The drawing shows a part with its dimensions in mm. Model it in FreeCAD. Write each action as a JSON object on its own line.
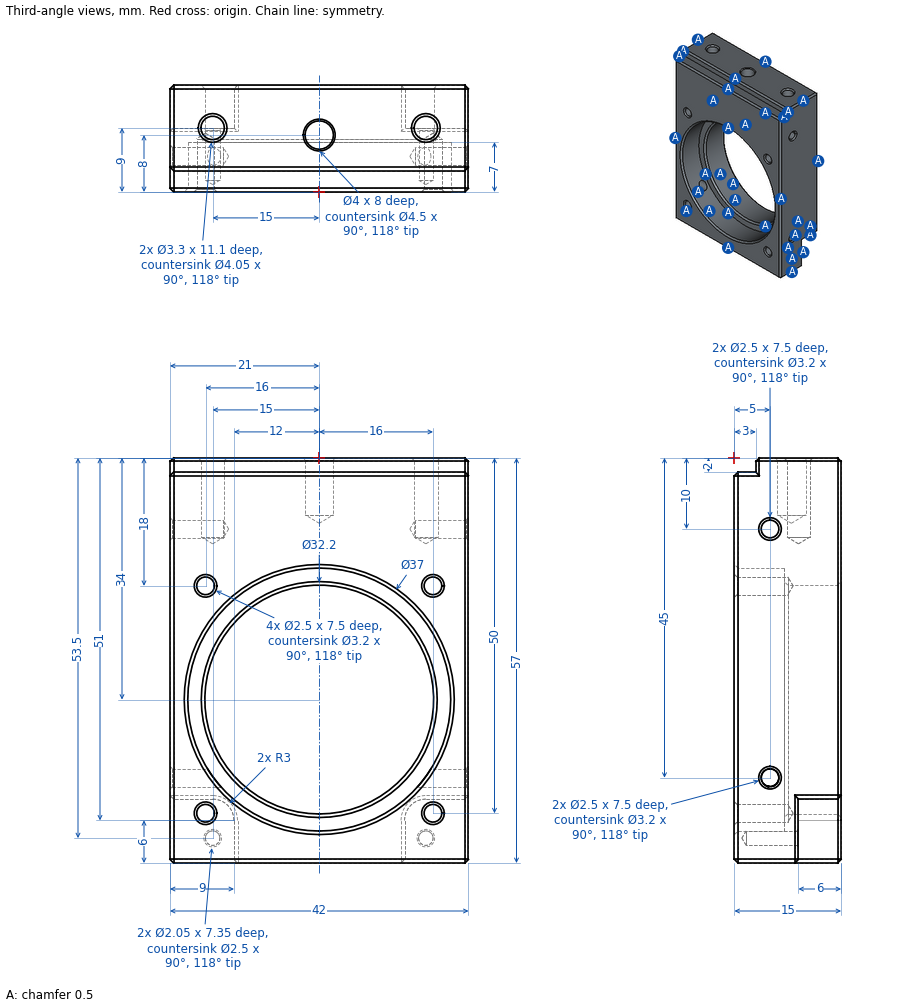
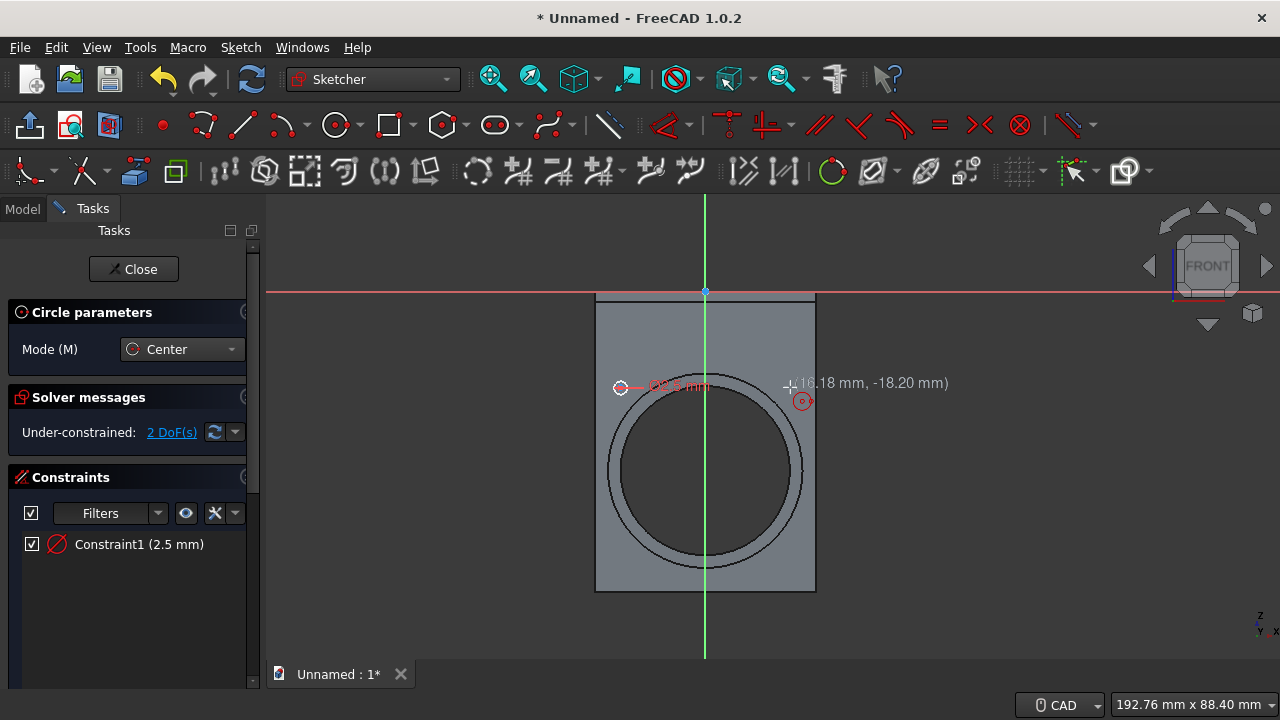
{"action": "left_click", "coordinate": [789, 387]}
{"action": "mouse_move", "coordinate": [794, 382]}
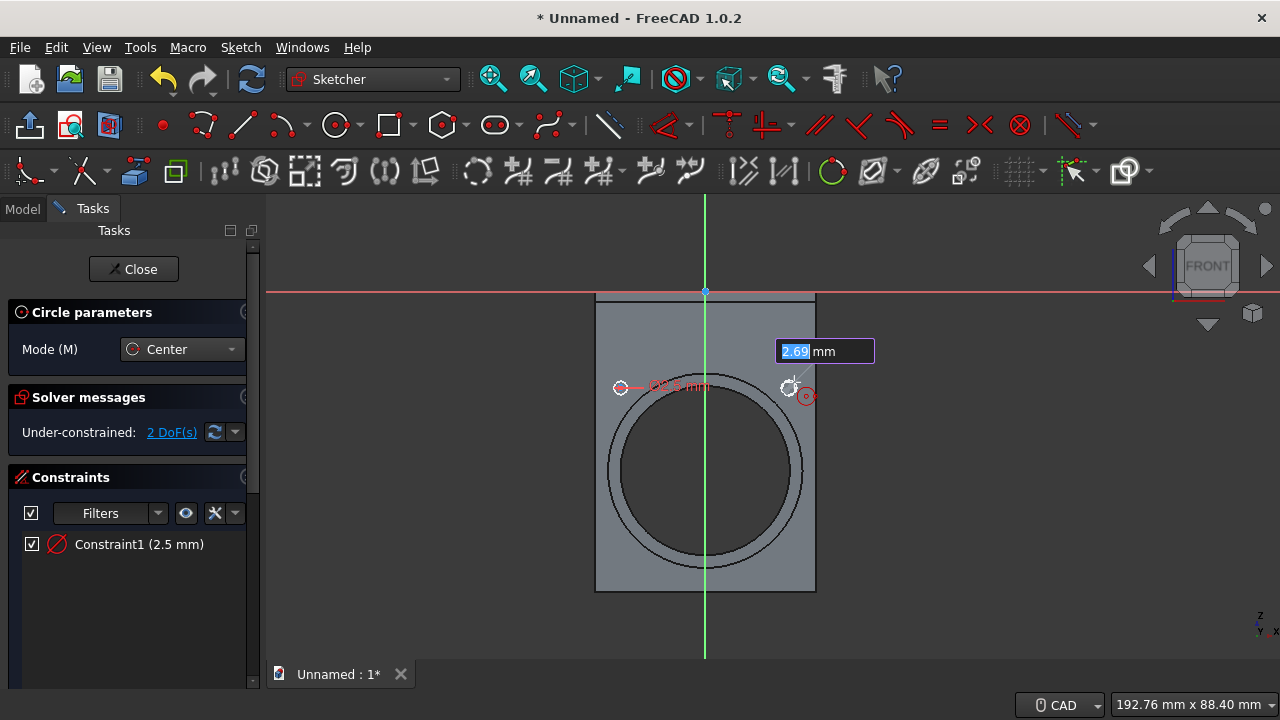
{"action": "type", "text": "2.5"}
{"action": "key", "text": "Return"}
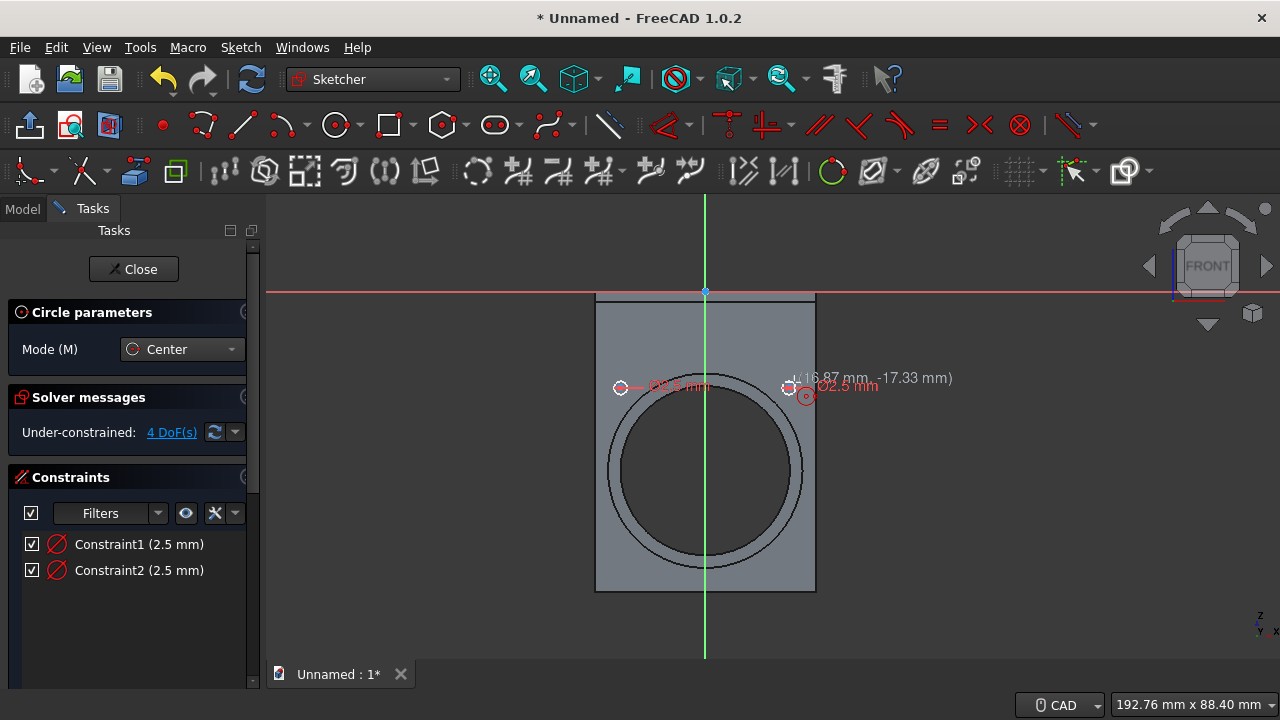
{"action": "scroll", "coordinate": [789, 555], "scroll_direction": "up", "scroll_amount": 7}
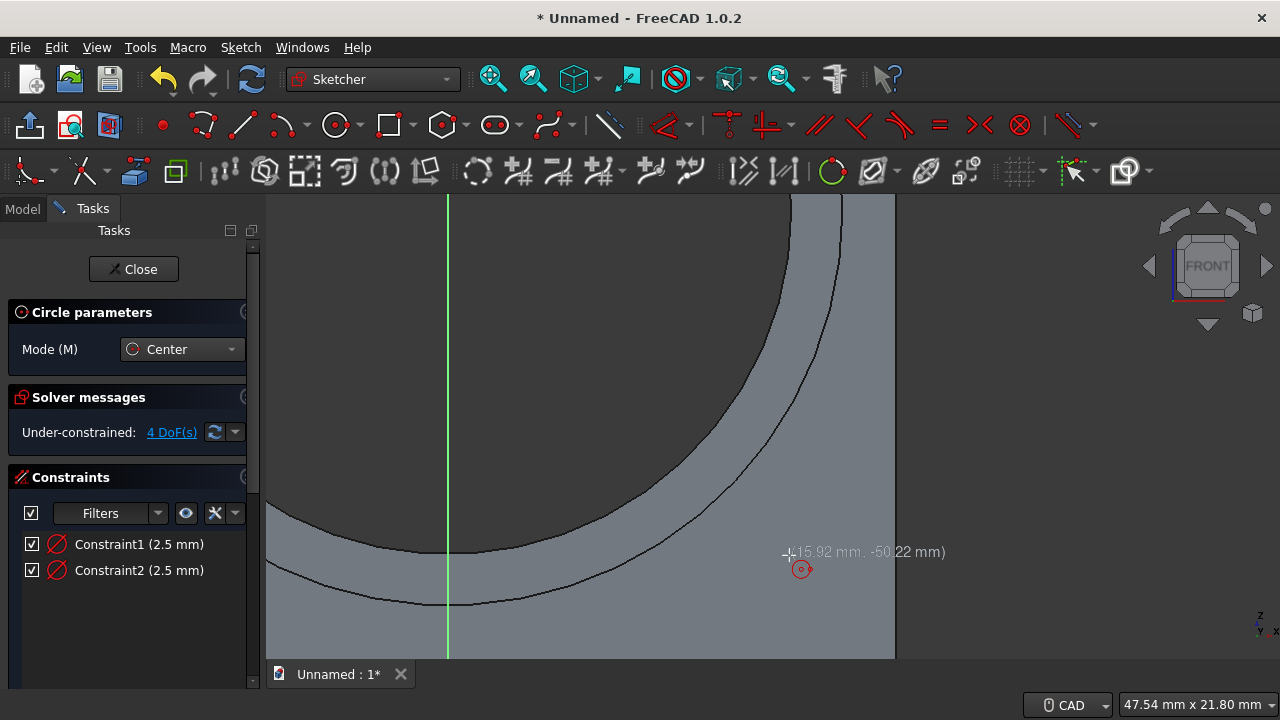
{"action": "scroll", "coordinate": [789, 556], "scroll_direction": "down", "scroll_amount": 7}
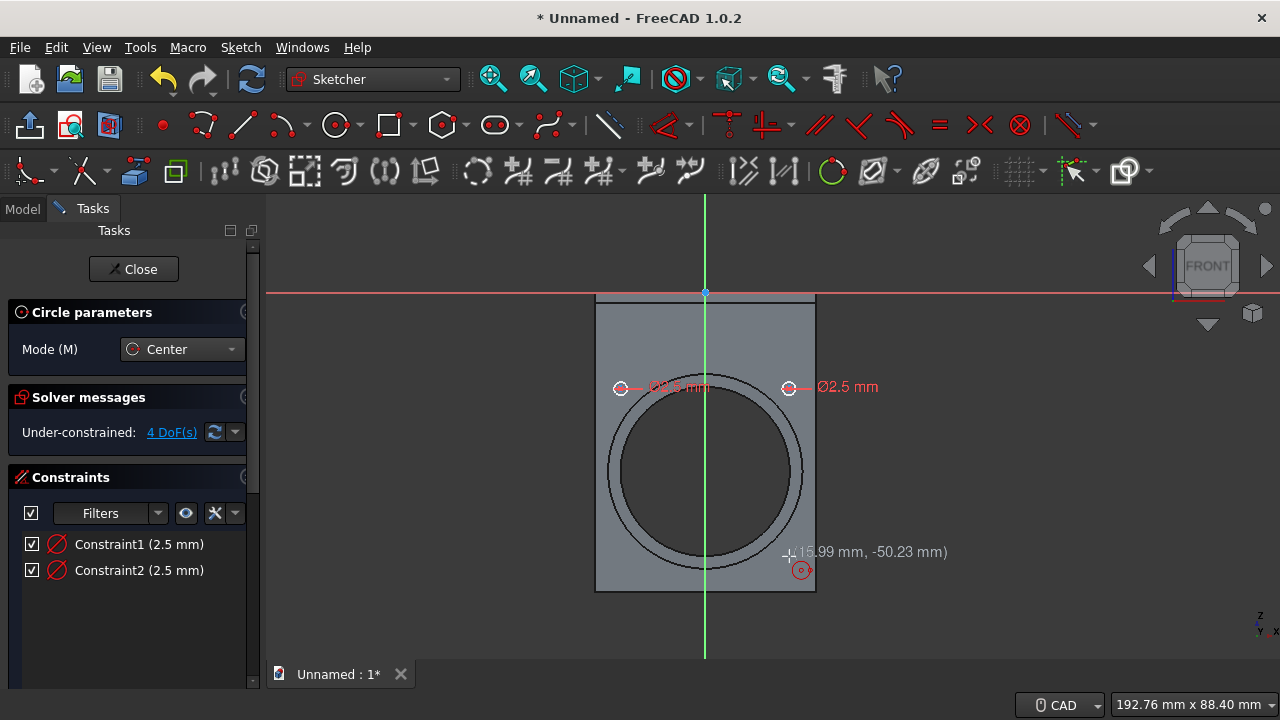
{"action": "left_click", "coordinate": [789, 556]}
{"action": "mouse_move", "coordinate": [794, 551]}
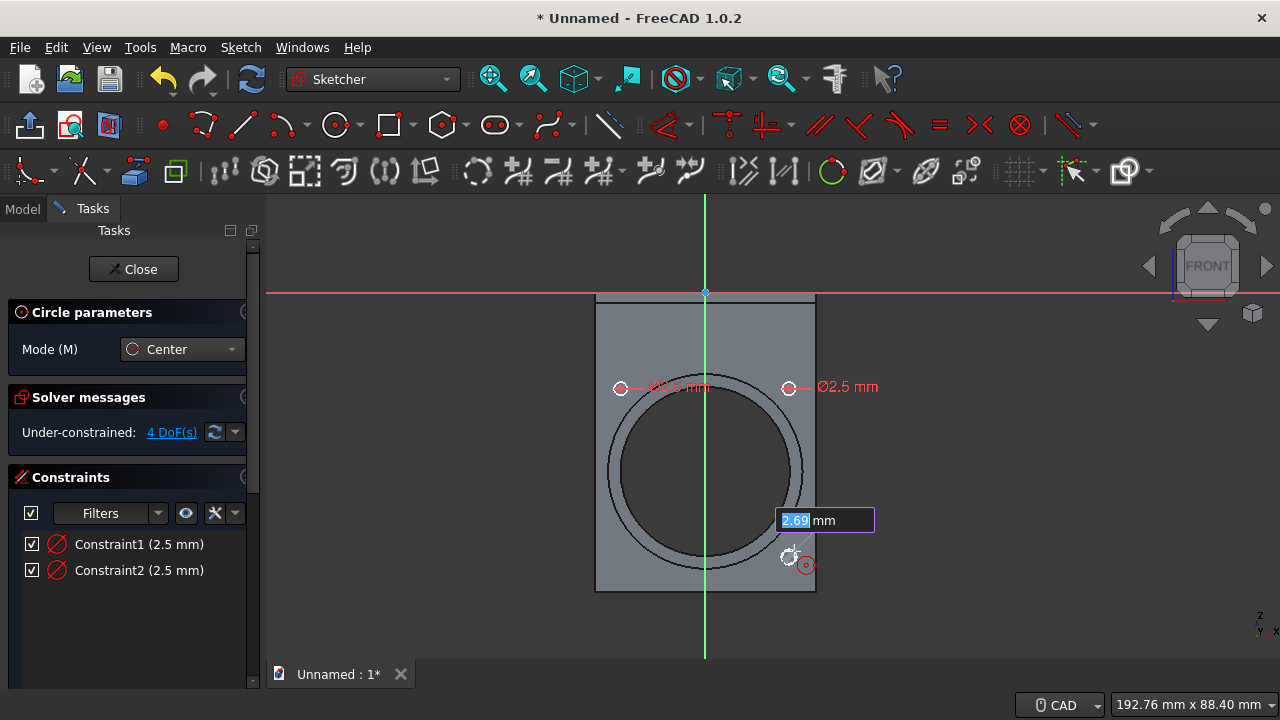
{"action": "type", "text": "2.5"}
{"action": "key", "text": "Return"}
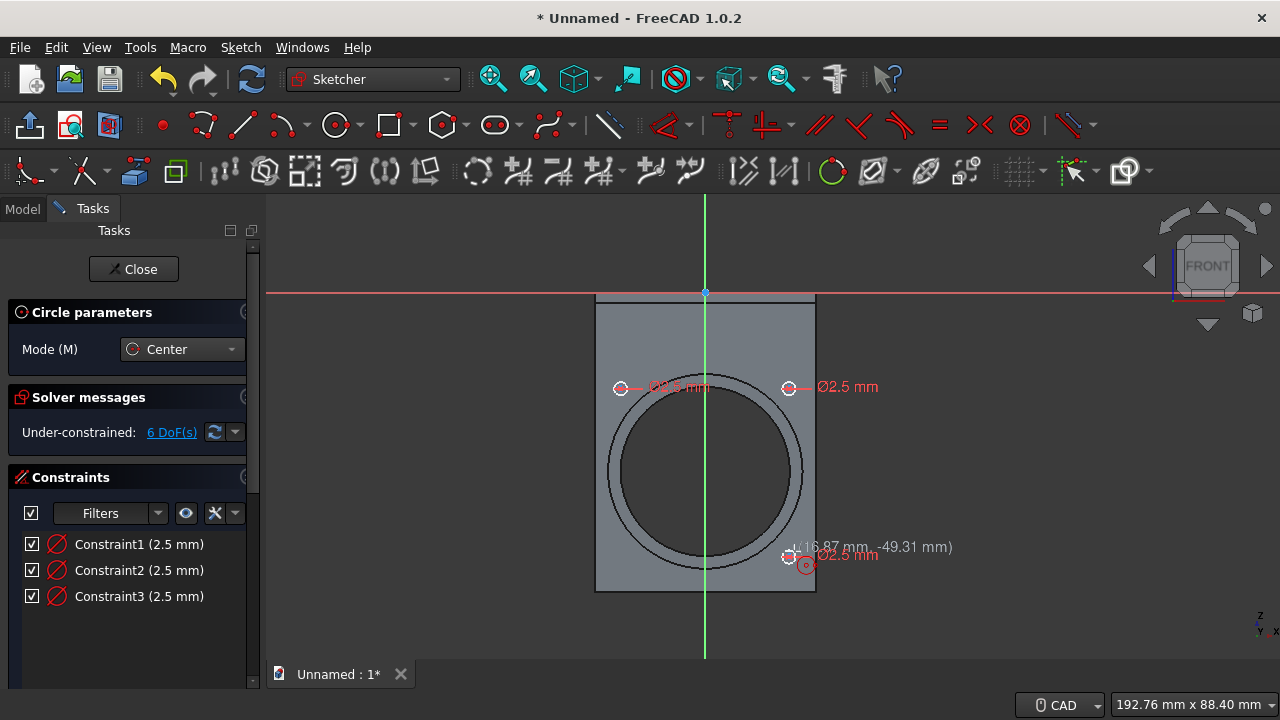
{"action": "scroll", "coordinate": [621, 556], "scroll_direction": "up", "scroll_amount": 7}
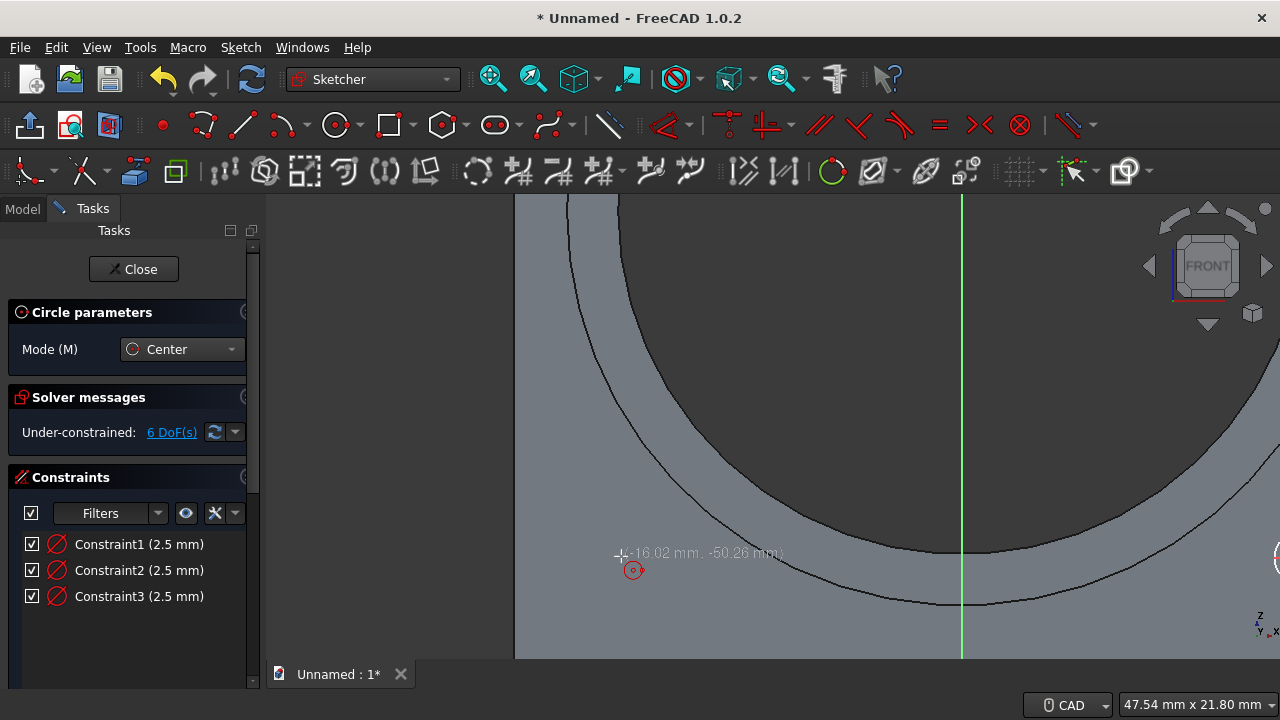
{"action": "scroll", "coordinate": [620, 556], "scroll_direction": "down", "scroll_amount": 7}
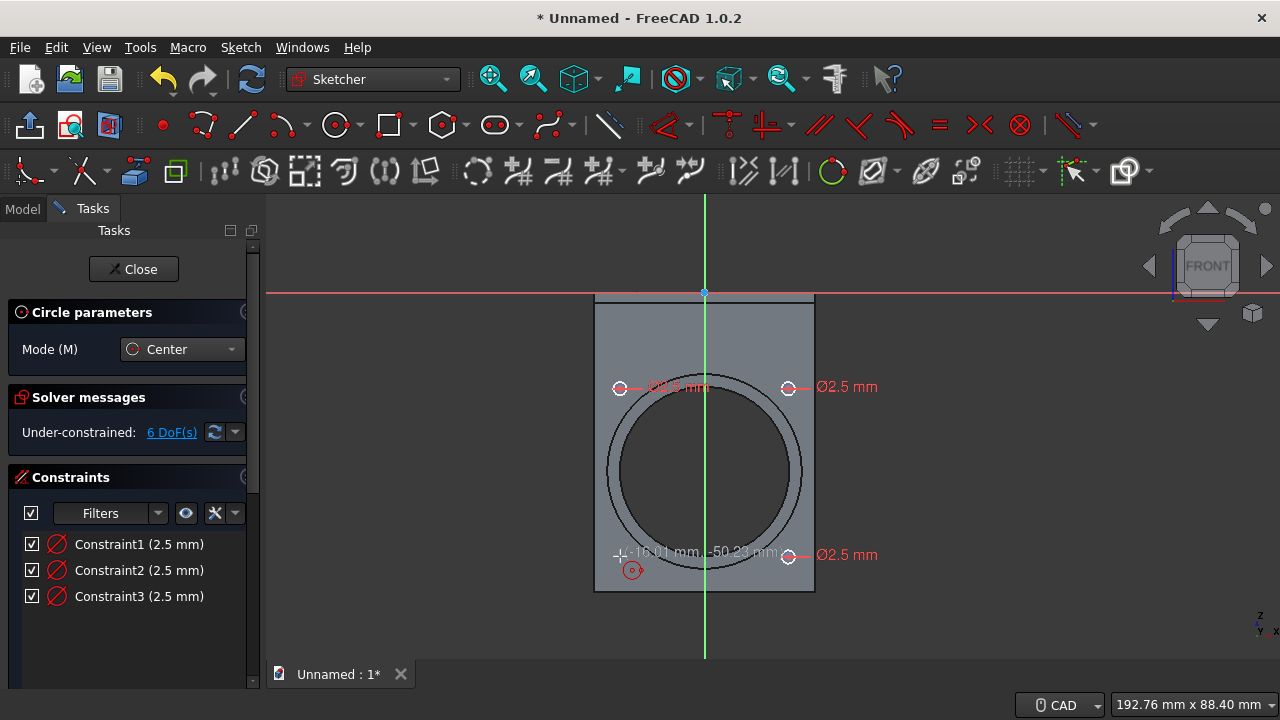
{"action": "left_click", "coordinate": [620, 556]}
{"action": "mouse_move", "coordinate": [625, 551]}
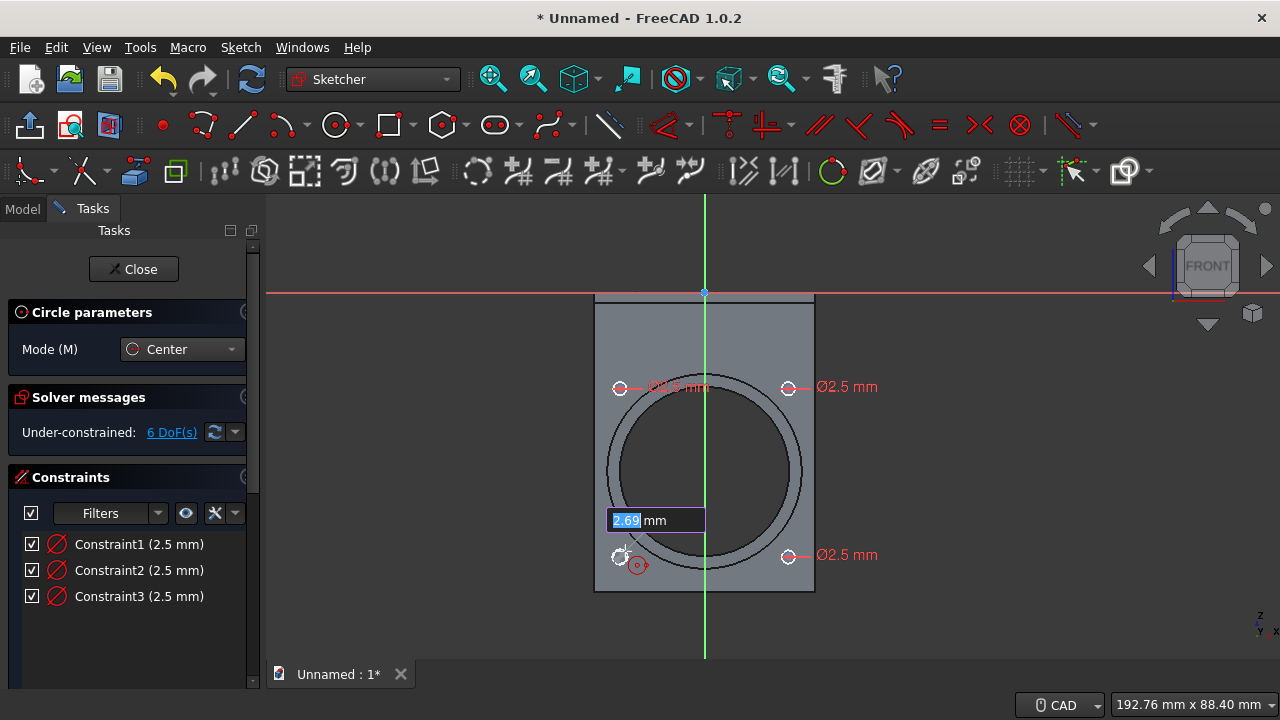
{"action": "type", "text": "2.5"}
{"action": "key", "text": "Return"}
{"action": "key", "text": "Escape"}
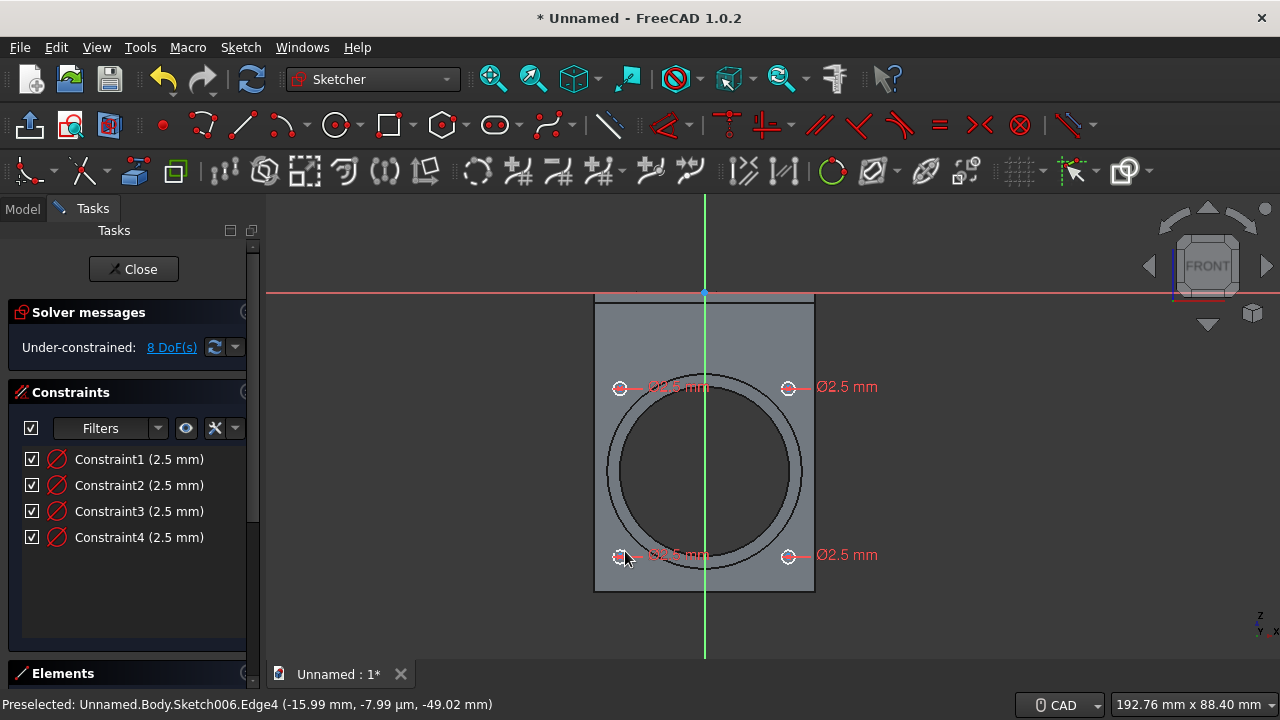
{"action": "left_click", "coordinate": [620, 389]}